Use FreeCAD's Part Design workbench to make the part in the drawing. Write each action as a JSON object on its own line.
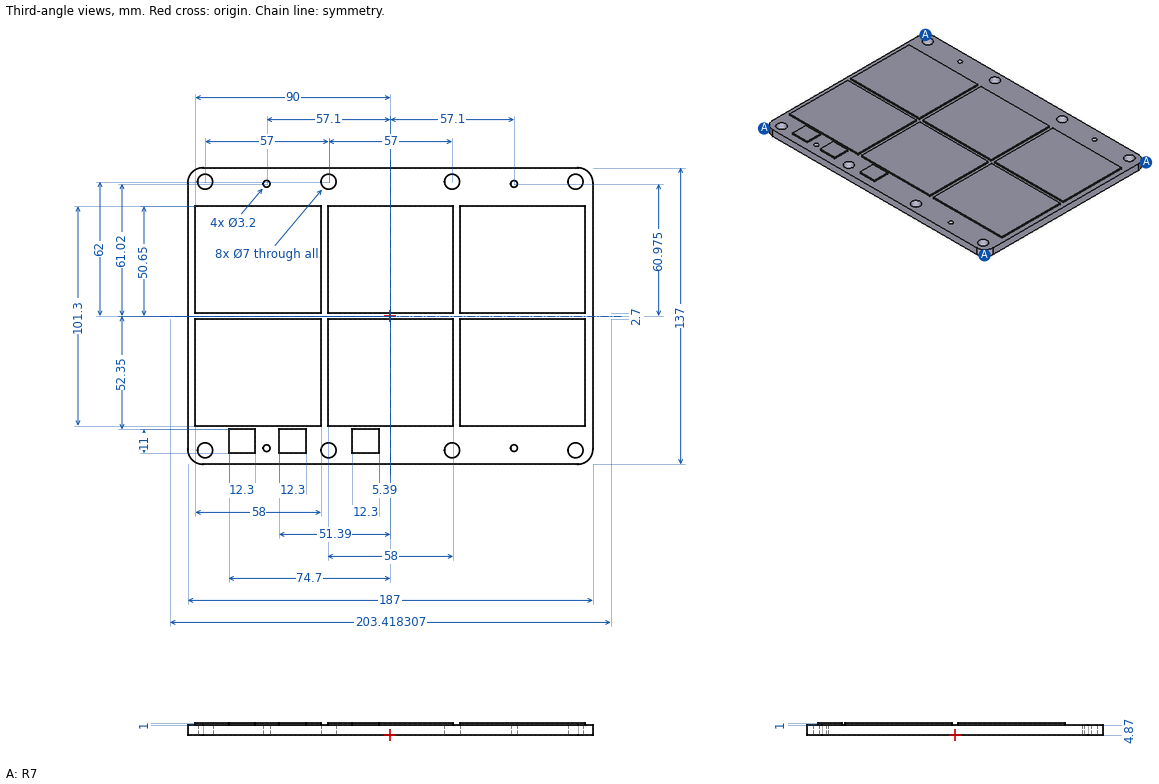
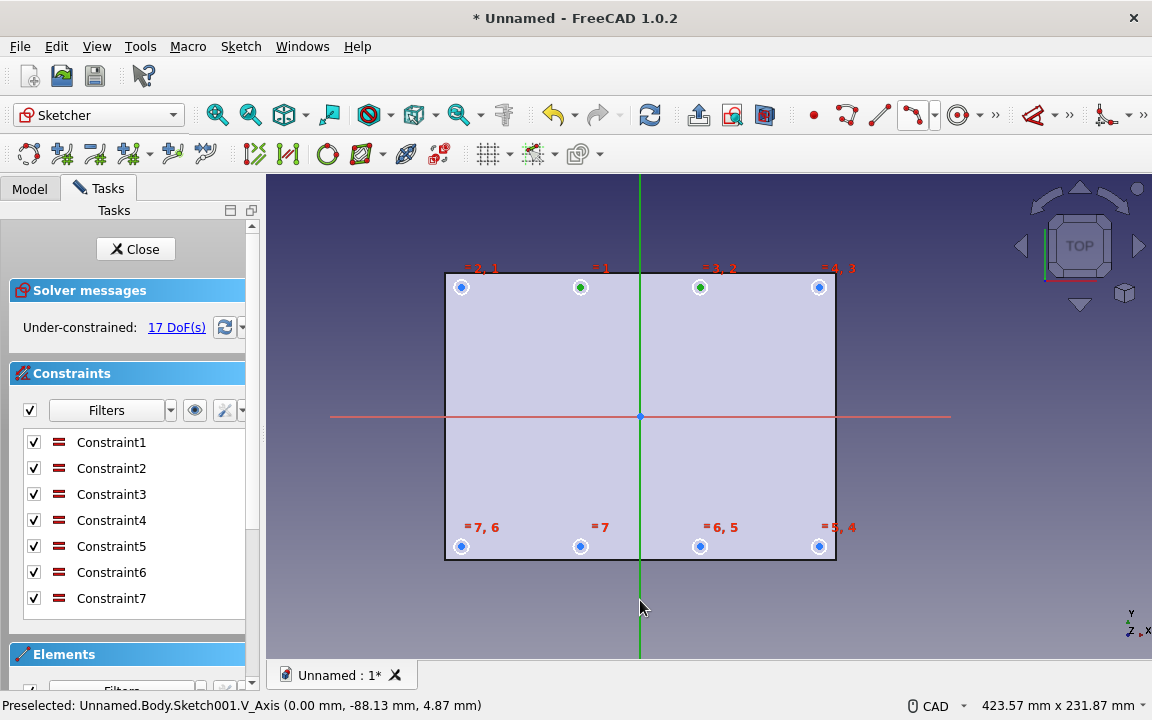
{"action": "key", "text": "s"}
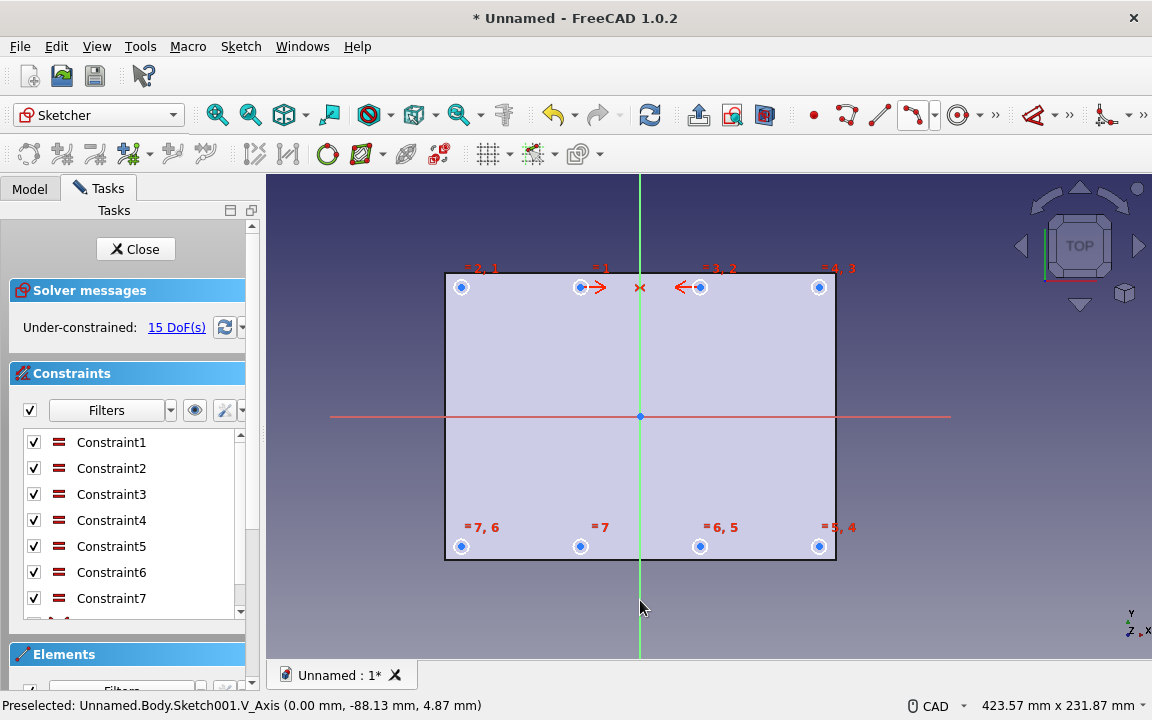
{"action": "left_click", "coordinate": [462, 287]}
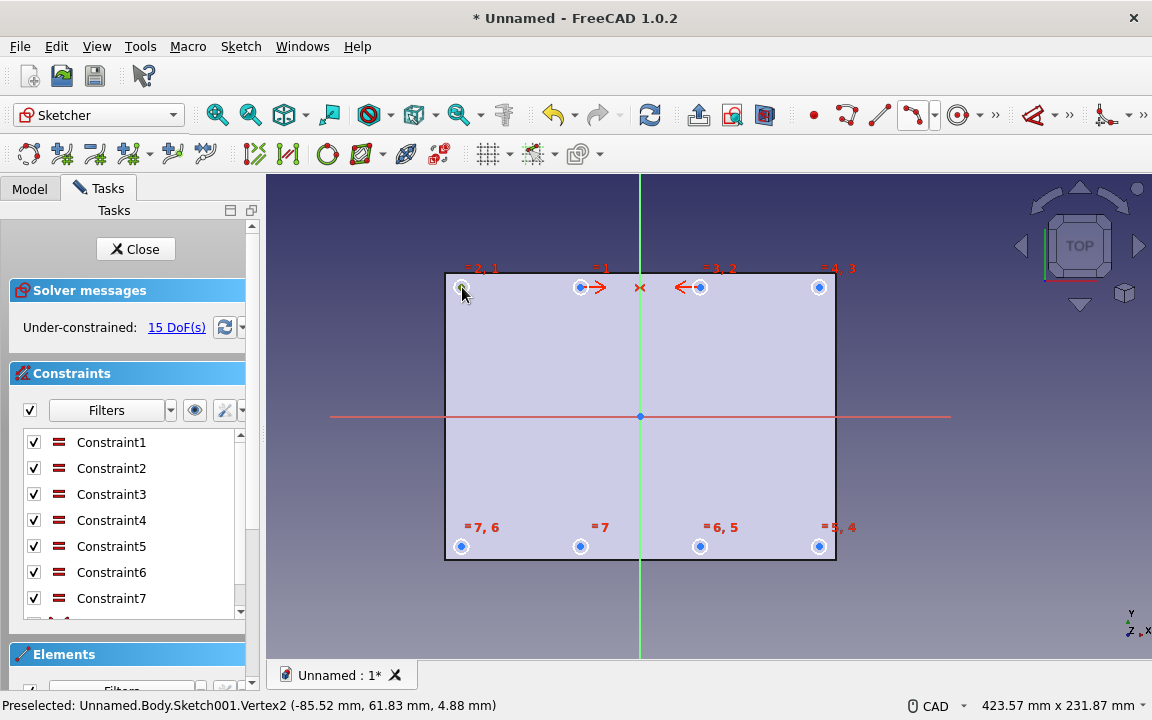
{"action": "left_click", "coordinate": [819, 287]}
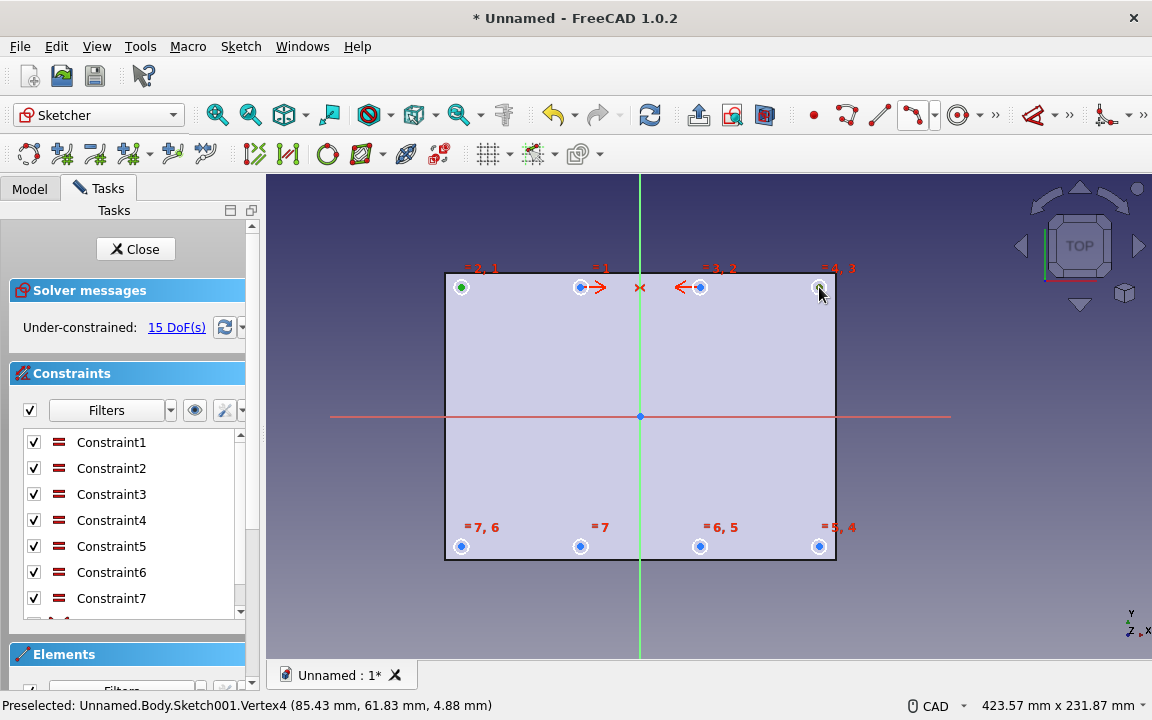
{"action": "left_click", "coordinate": [640, 600]}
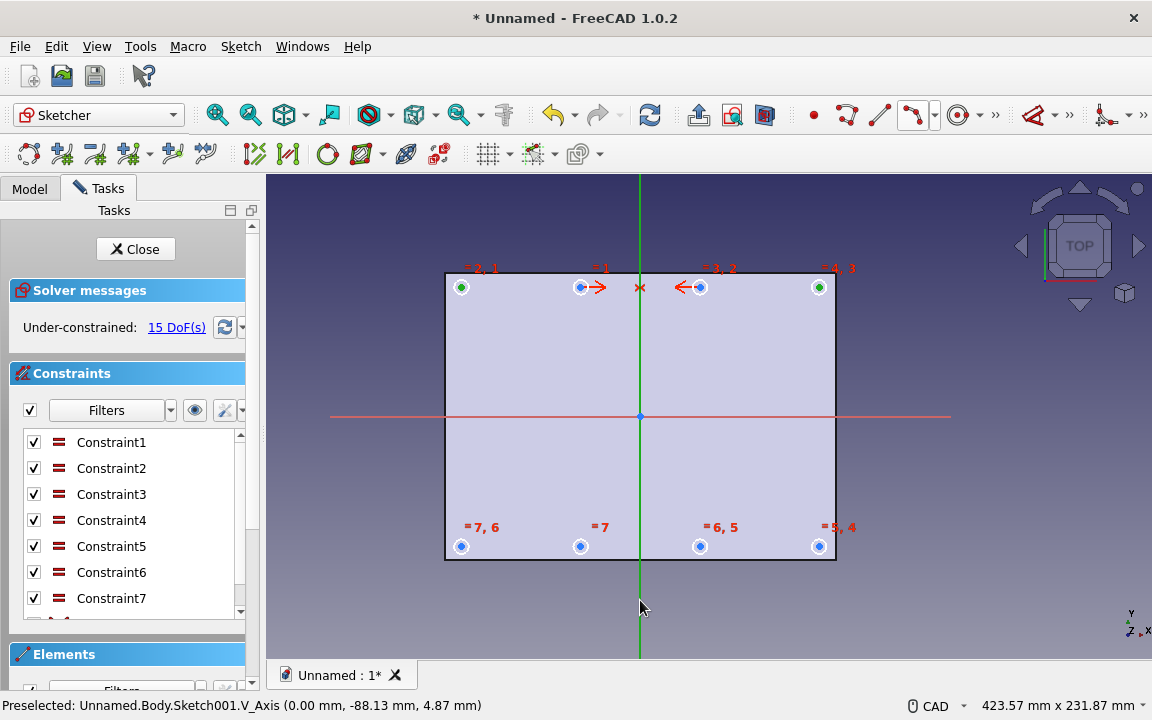
{"action": "key", "text": "s"}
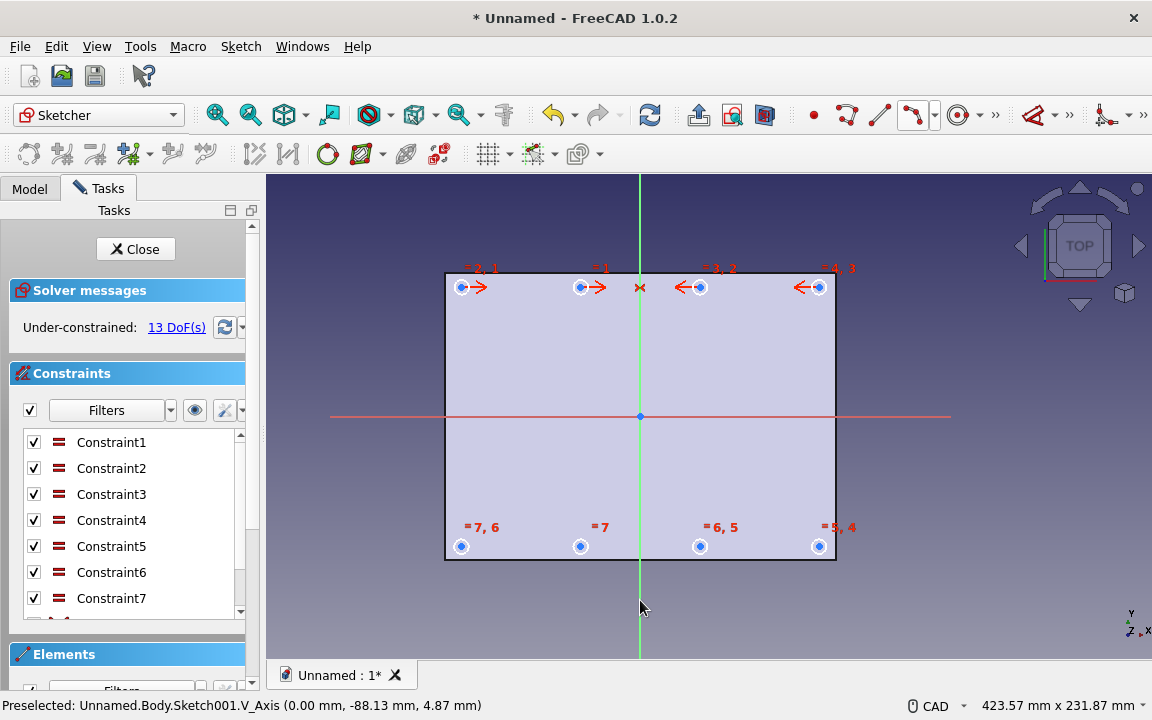
{"action": "left_click", "coordinate": [819, 287]}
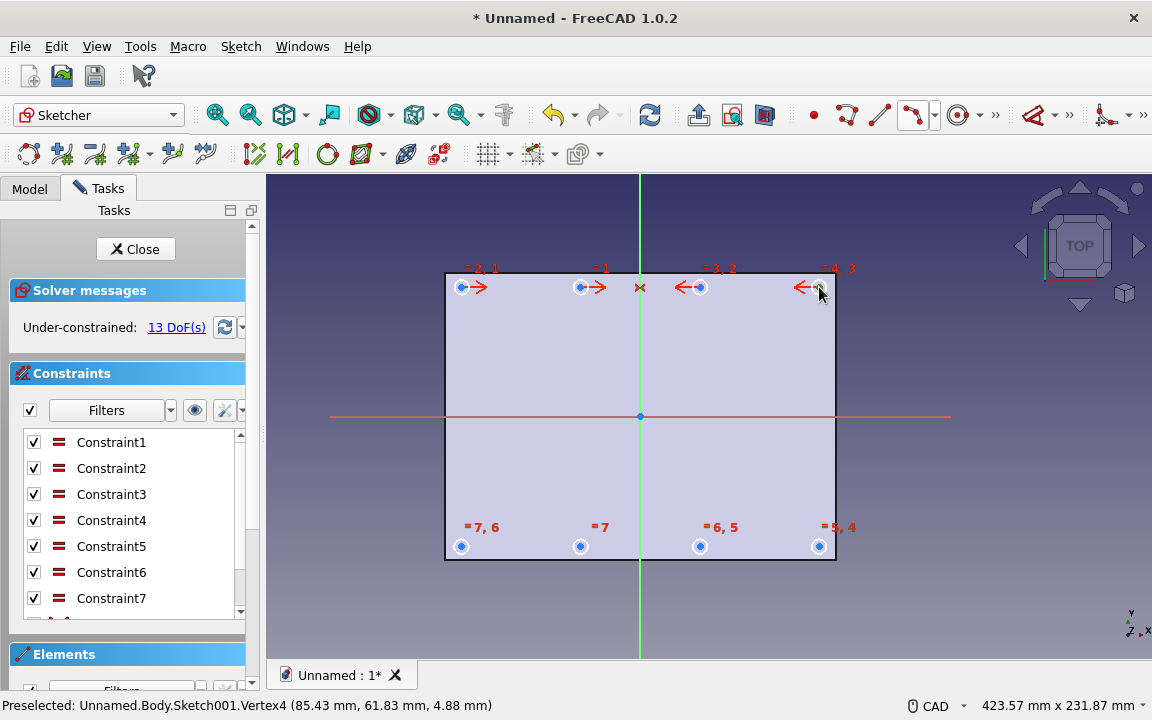
{"action": "left_click", "coordinate": [819, 547]}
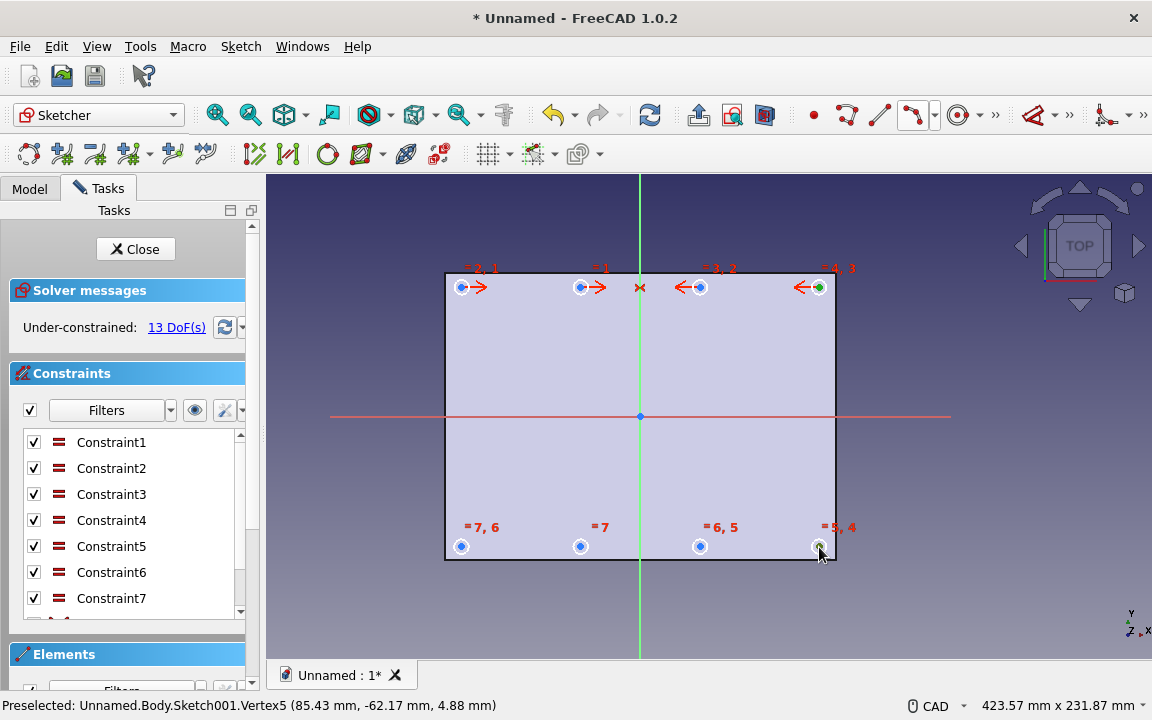
{"action": "left_click", "coordinate": [344, 417]}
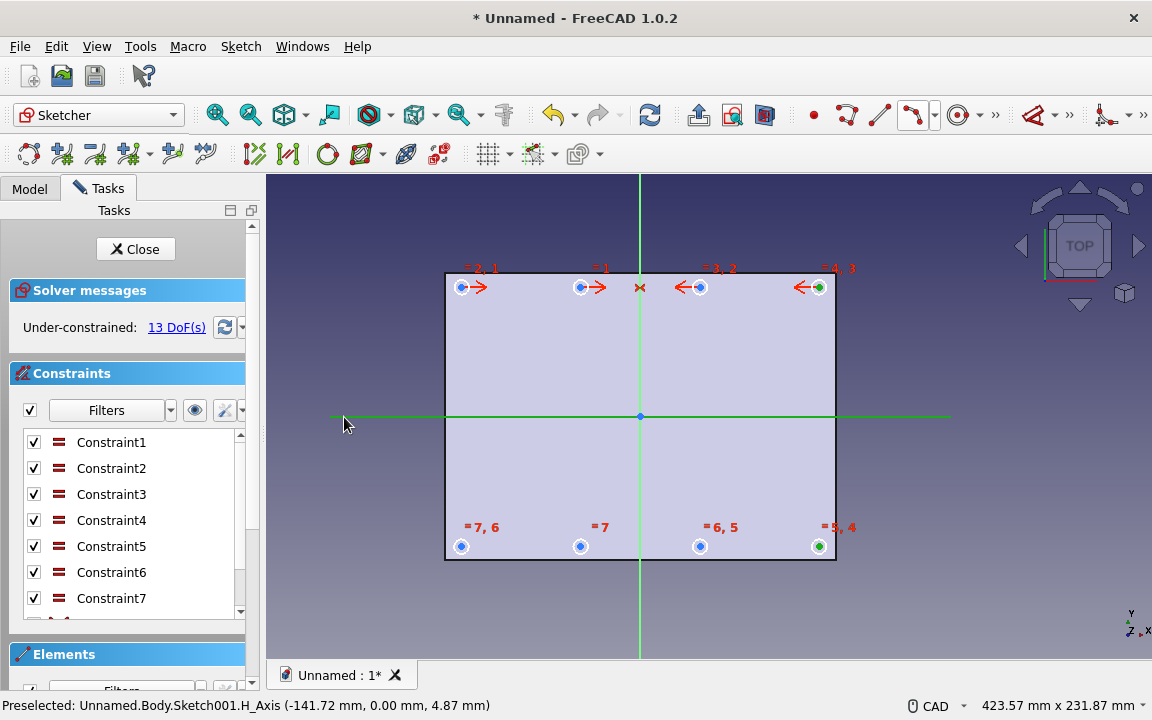
{"action": "key", "text": "s"}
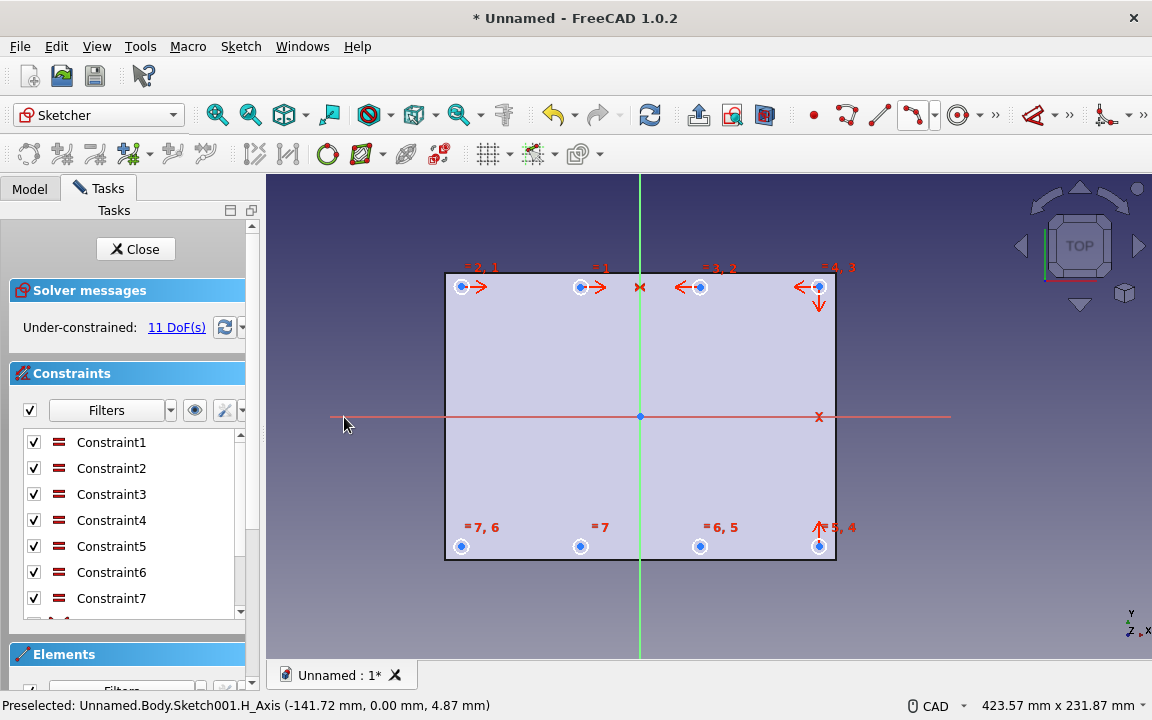
{"action": "left_click", "coordinate": [700, 287]}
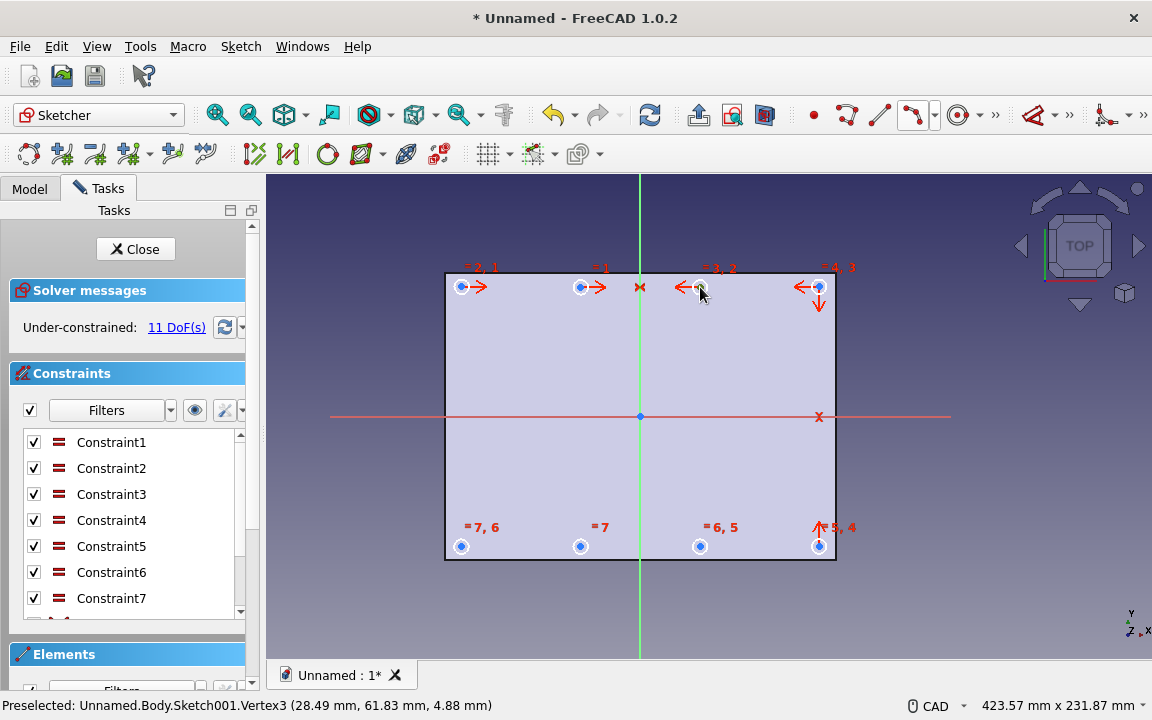
{"action": "left_click", "coordinate": [700, 547]}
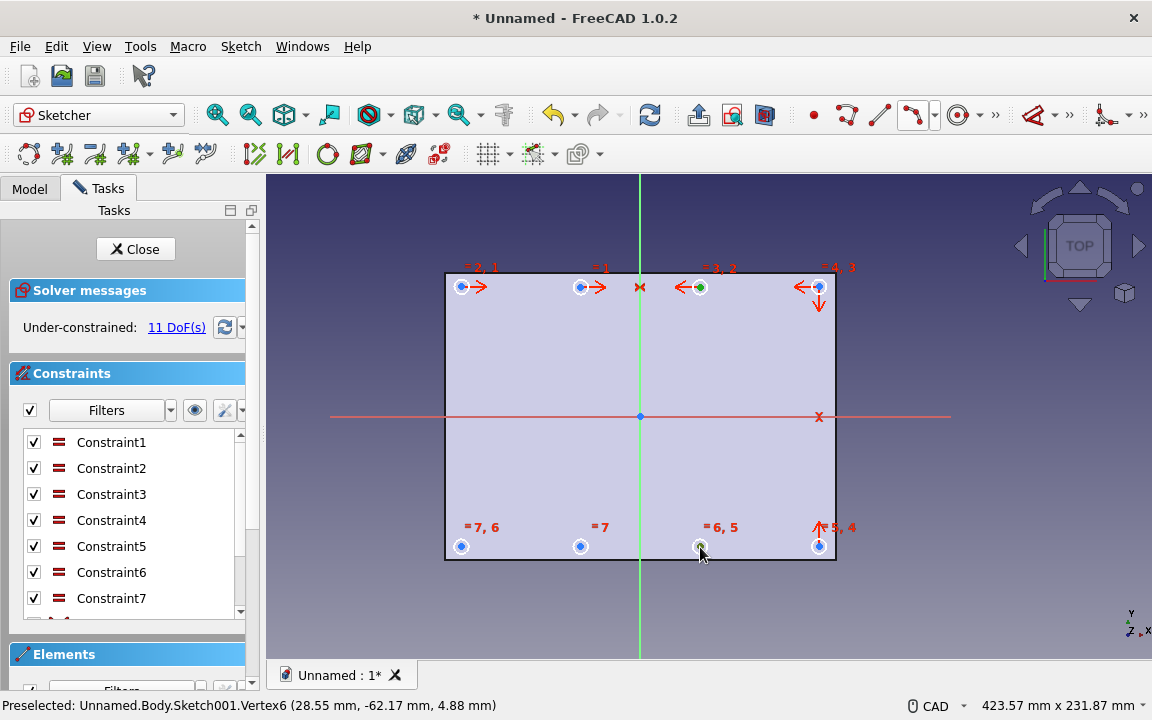
{"action": "left_click", "coordinate": [344, 417]}